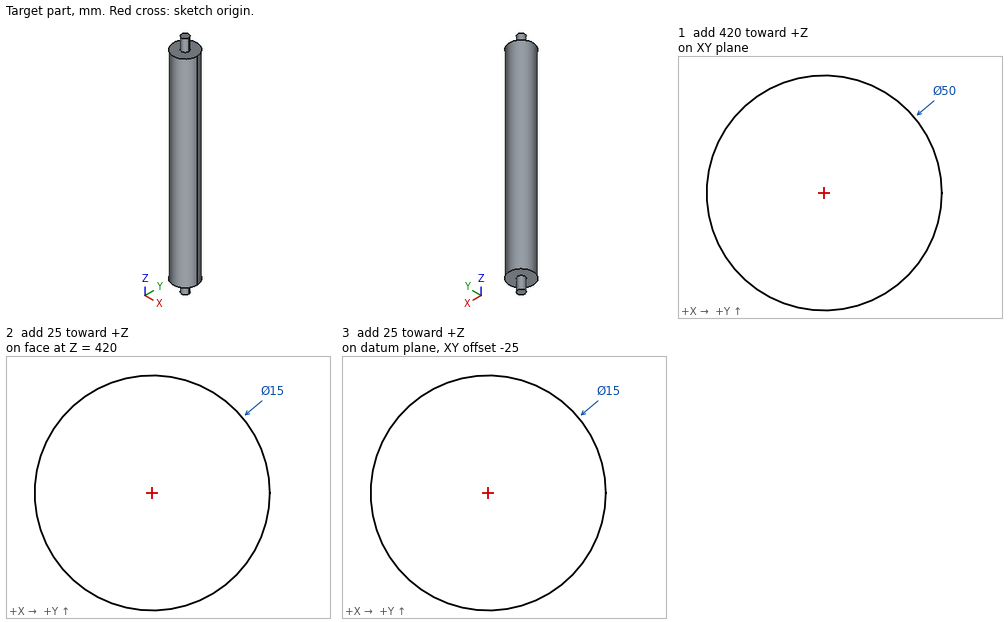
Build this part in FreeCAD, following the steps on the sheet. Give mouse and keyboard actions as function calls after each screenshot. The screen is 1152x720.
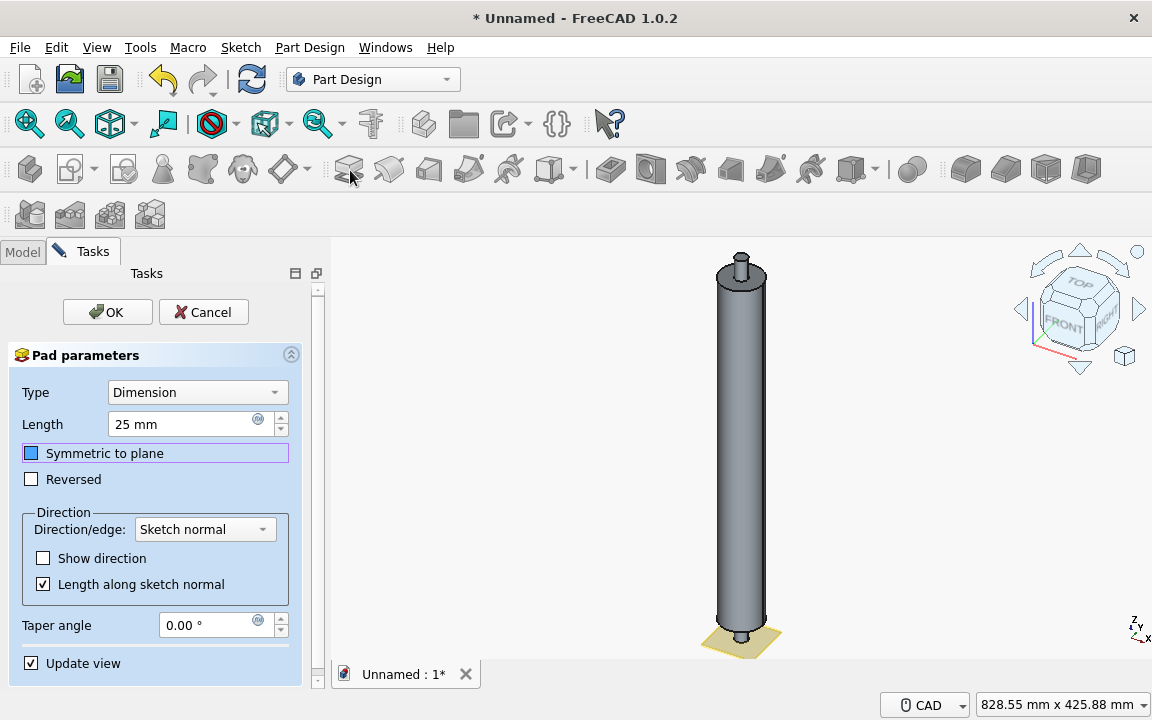
click(108, 312)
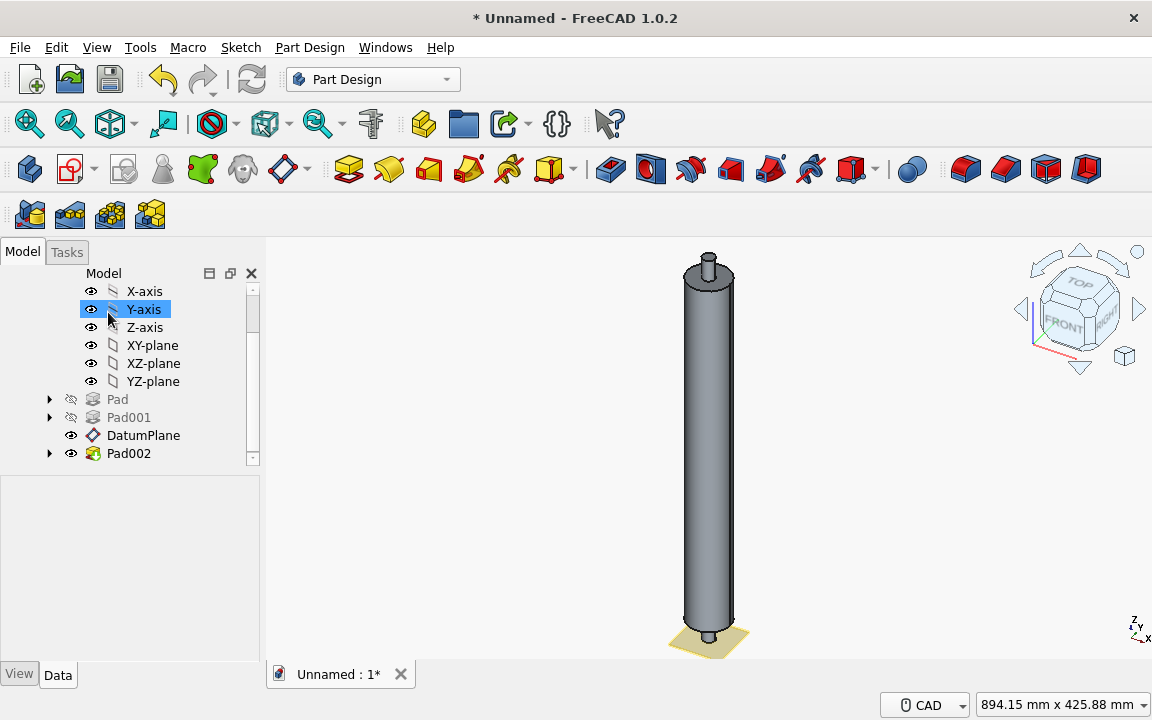
click(116, 435)
key(space)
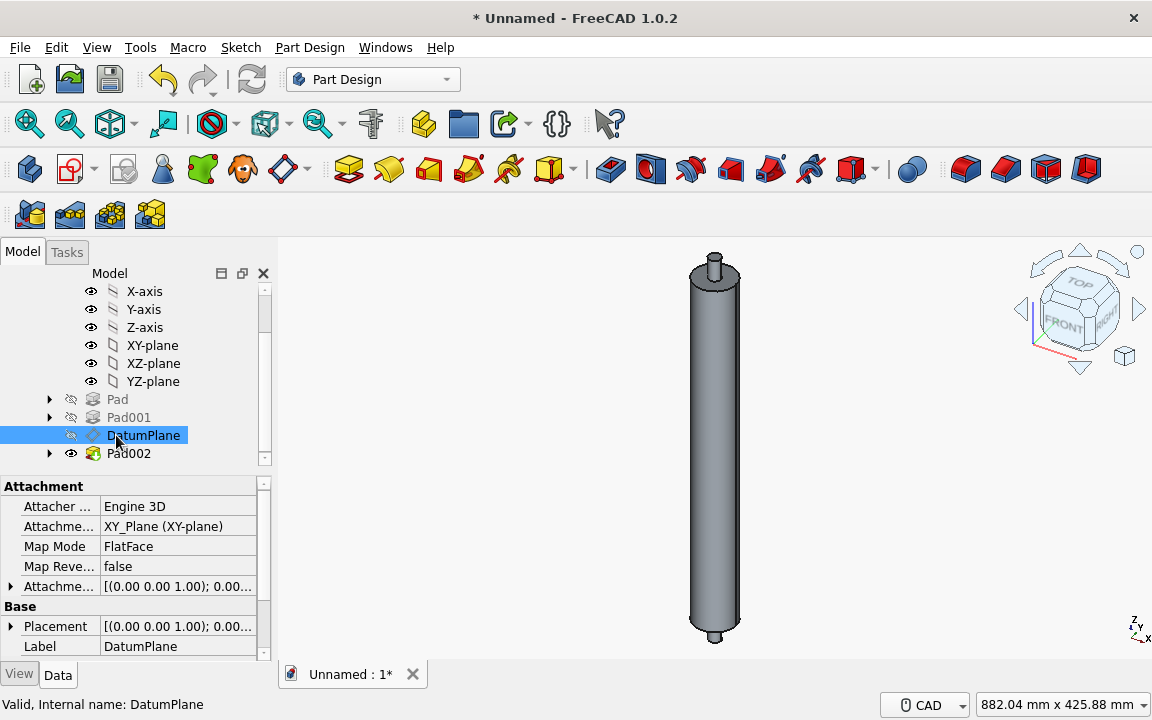
key(0)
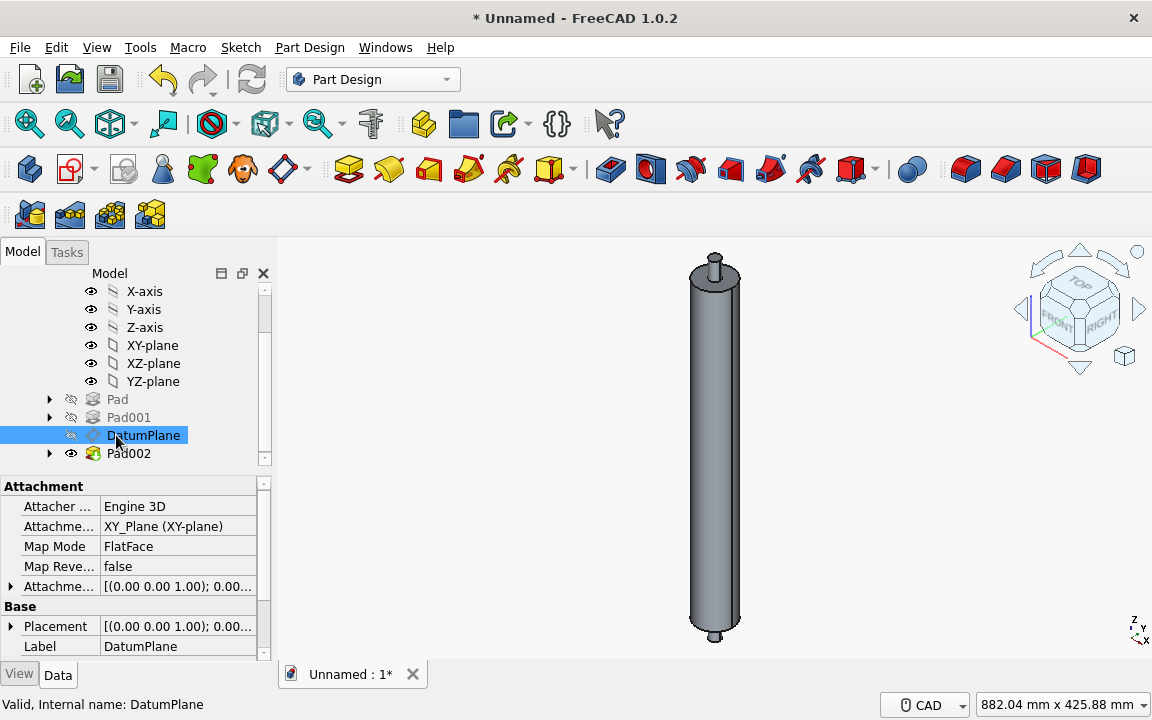
key(v)
key(f)